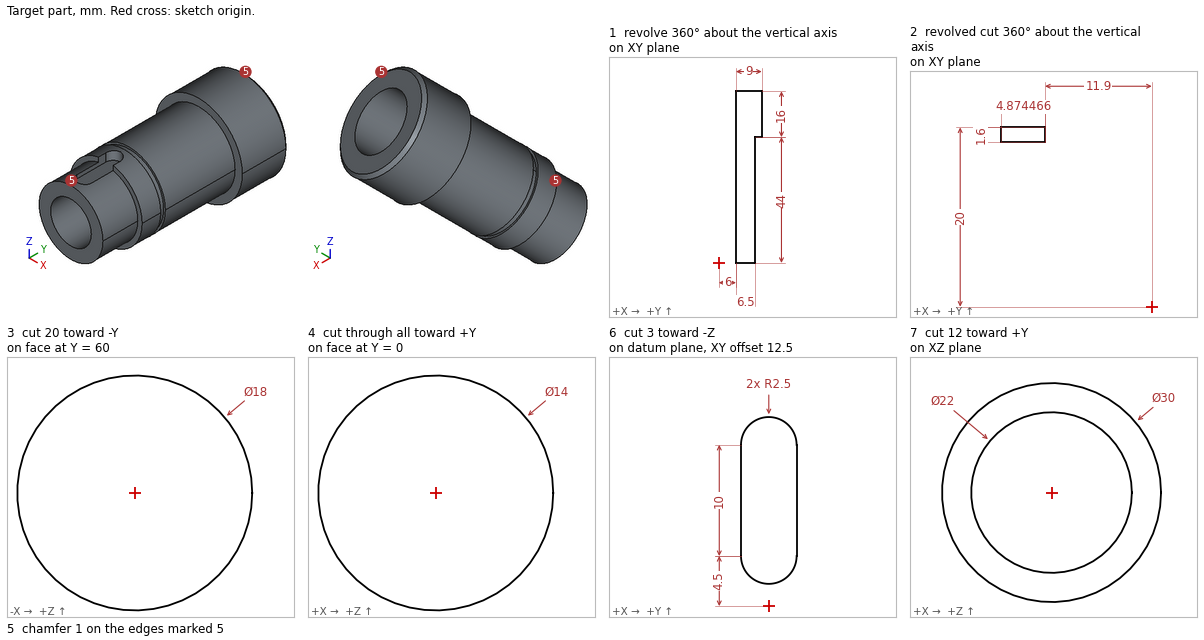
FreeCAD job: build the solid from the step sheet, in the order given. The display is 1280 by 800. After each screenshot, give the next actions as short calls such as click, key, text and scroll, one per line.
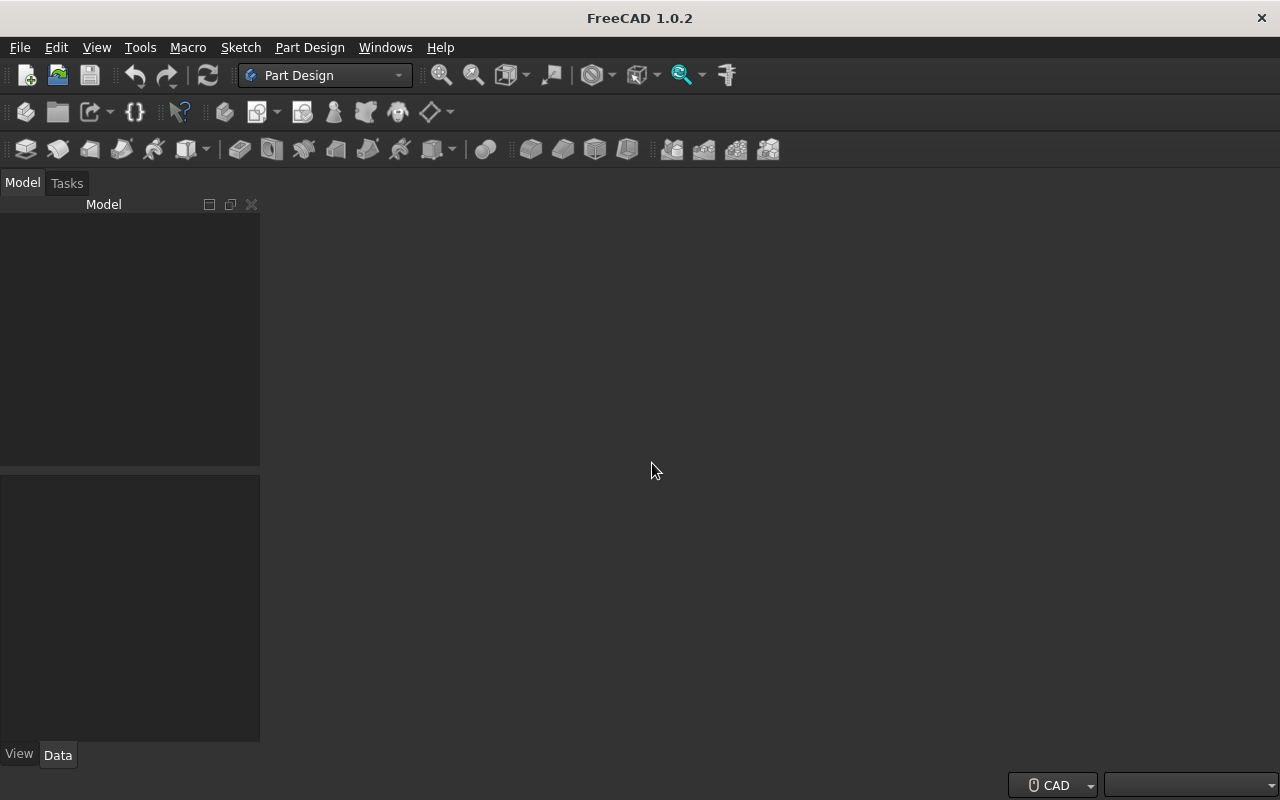
click(26, 76)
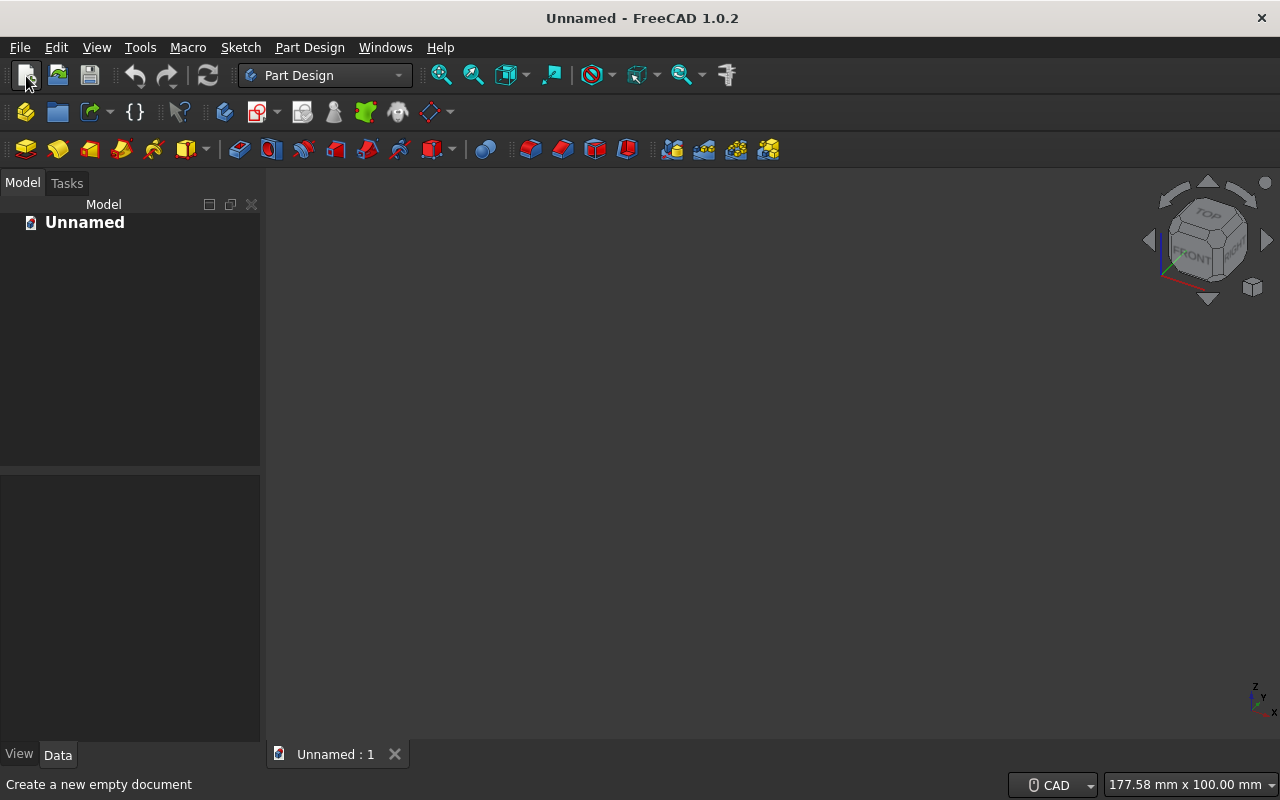
click(258, 112)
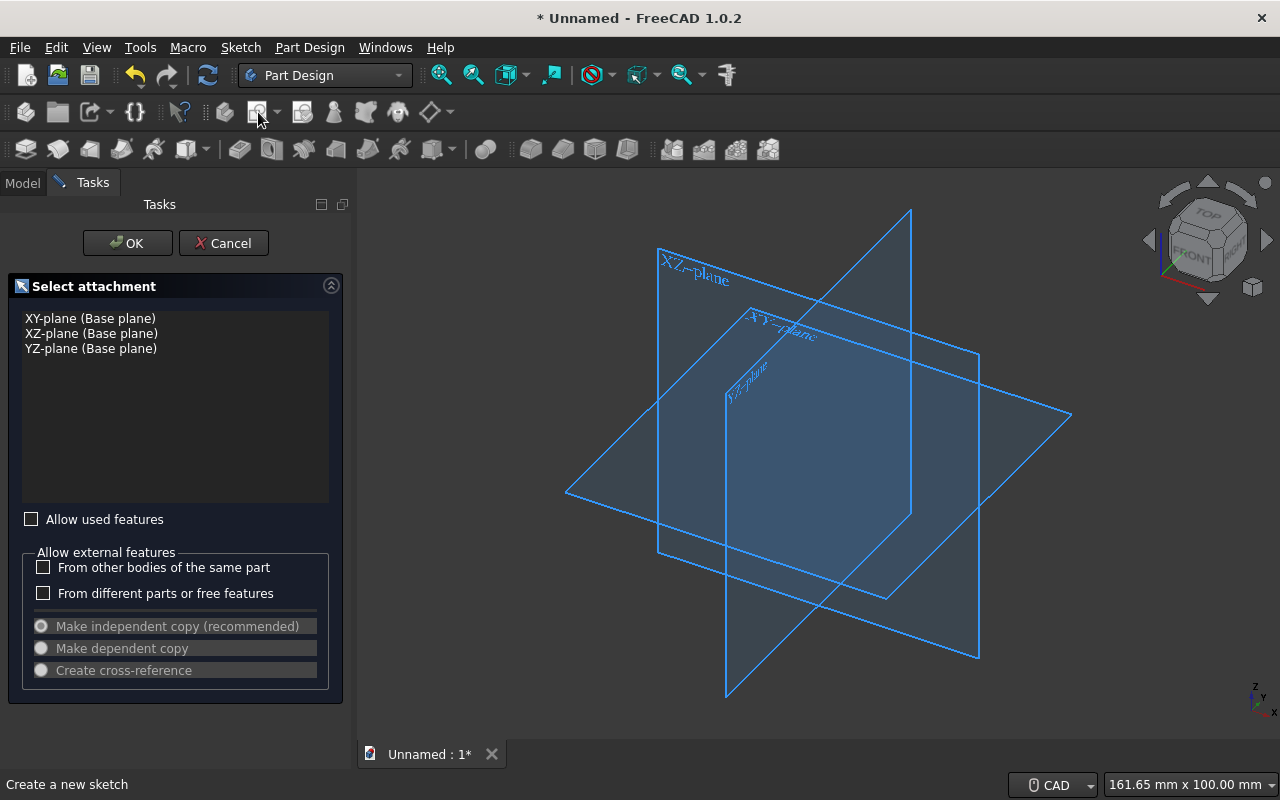
click(82, 318)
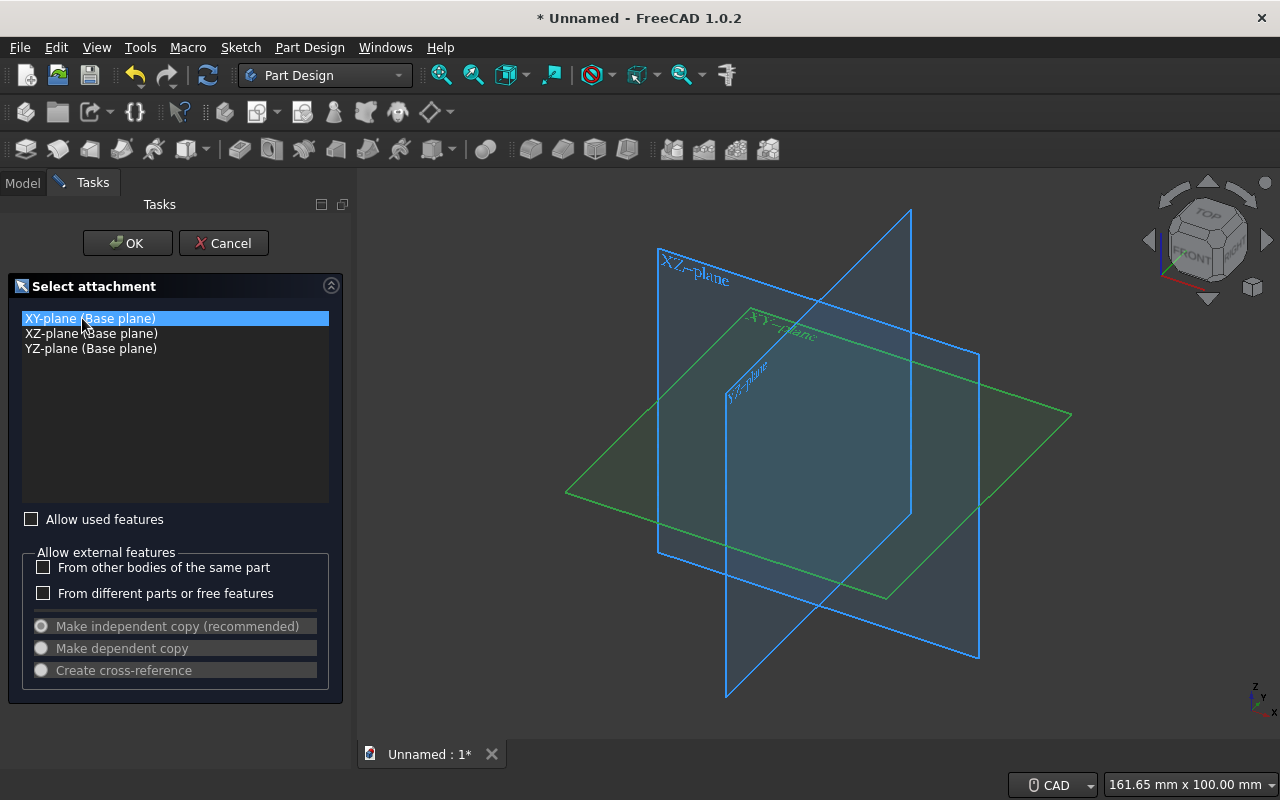
click(128, 243)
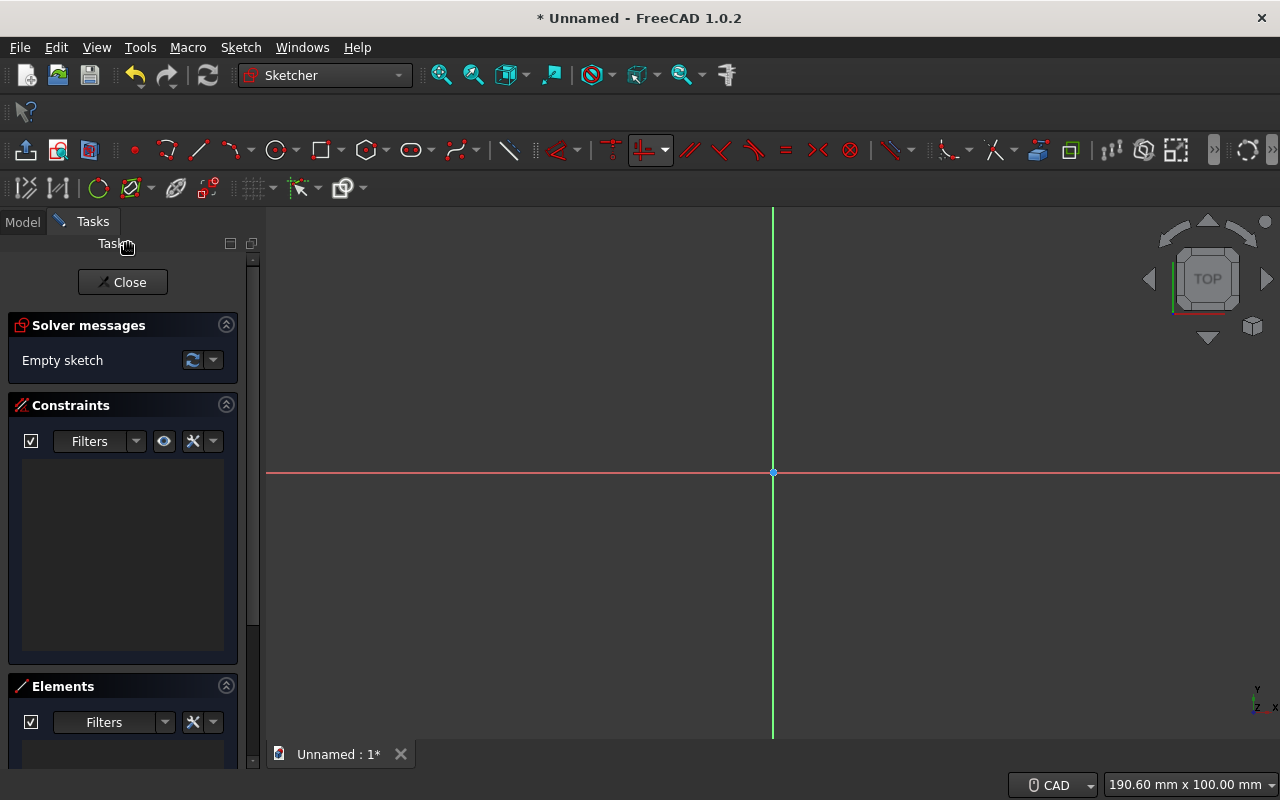
scroll(484, 711, down, 2)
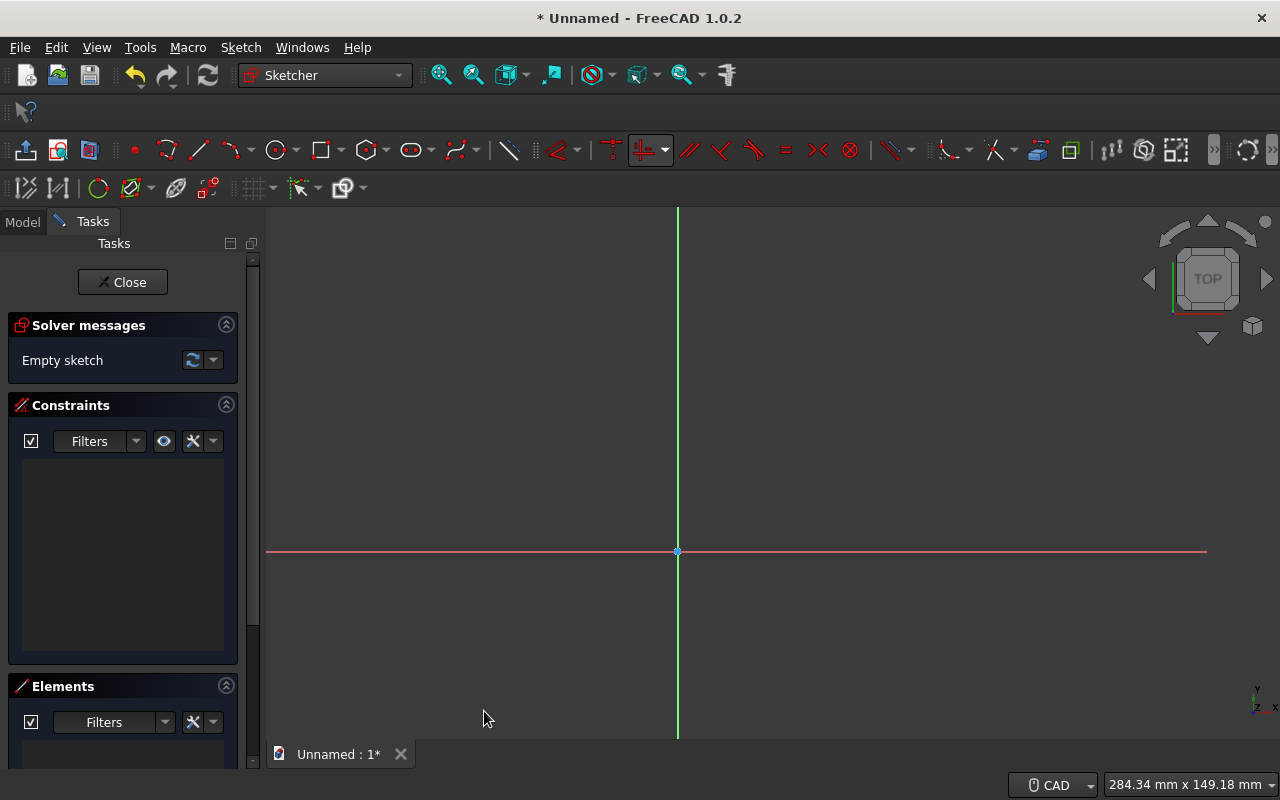
scroll(705, 387, up, 2)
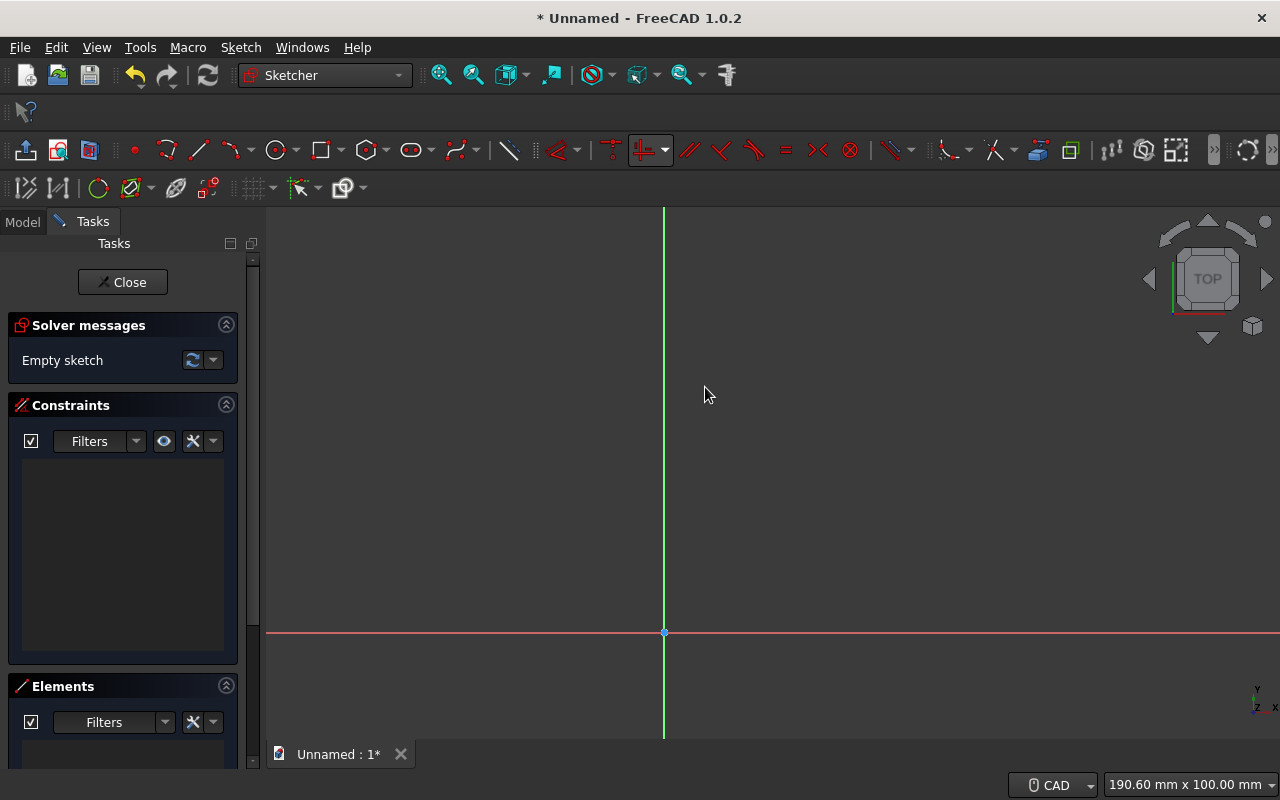
click(168, 150)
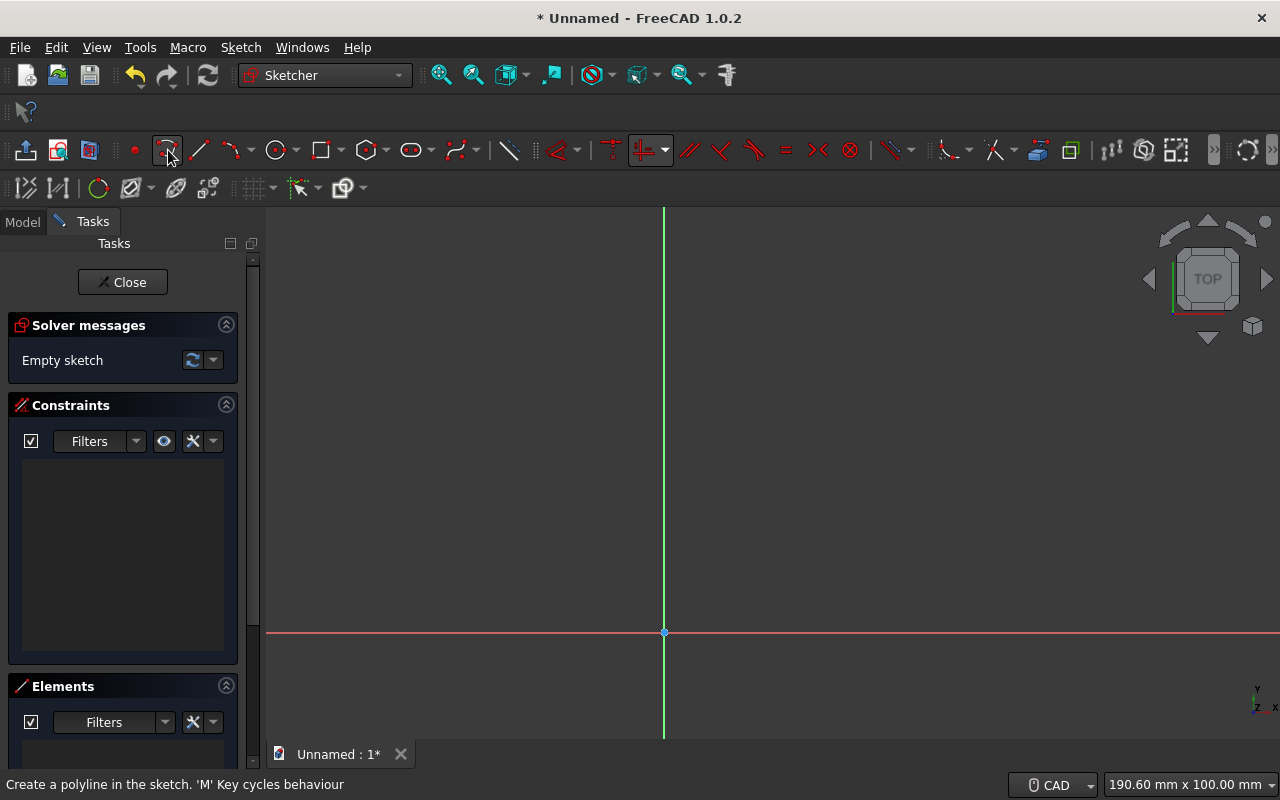
click(696, 633)
click(731, 624)
click(731, 399)
click(744, 399)
click(744, 313)
click(696, 313)
click(696, 633)
key(Escape)
key(Escape)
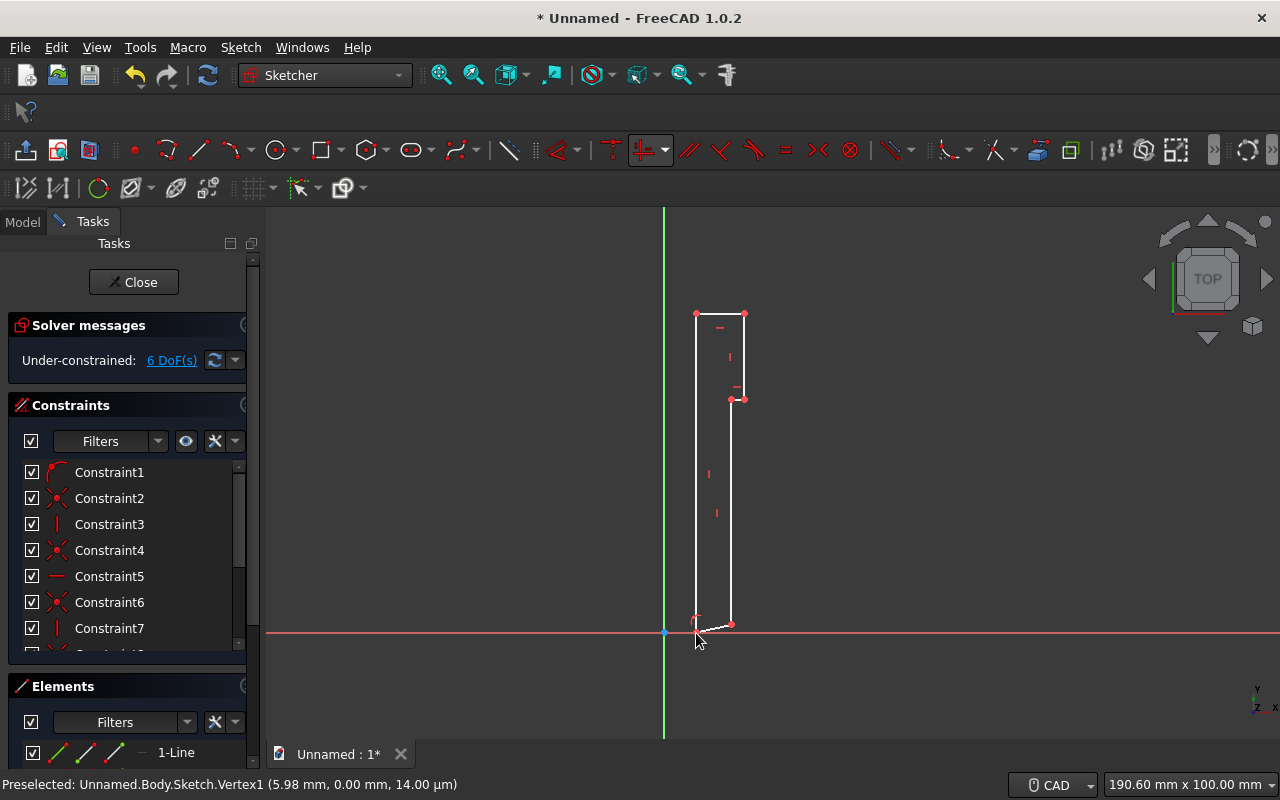
scroll(707, 630, up, 2)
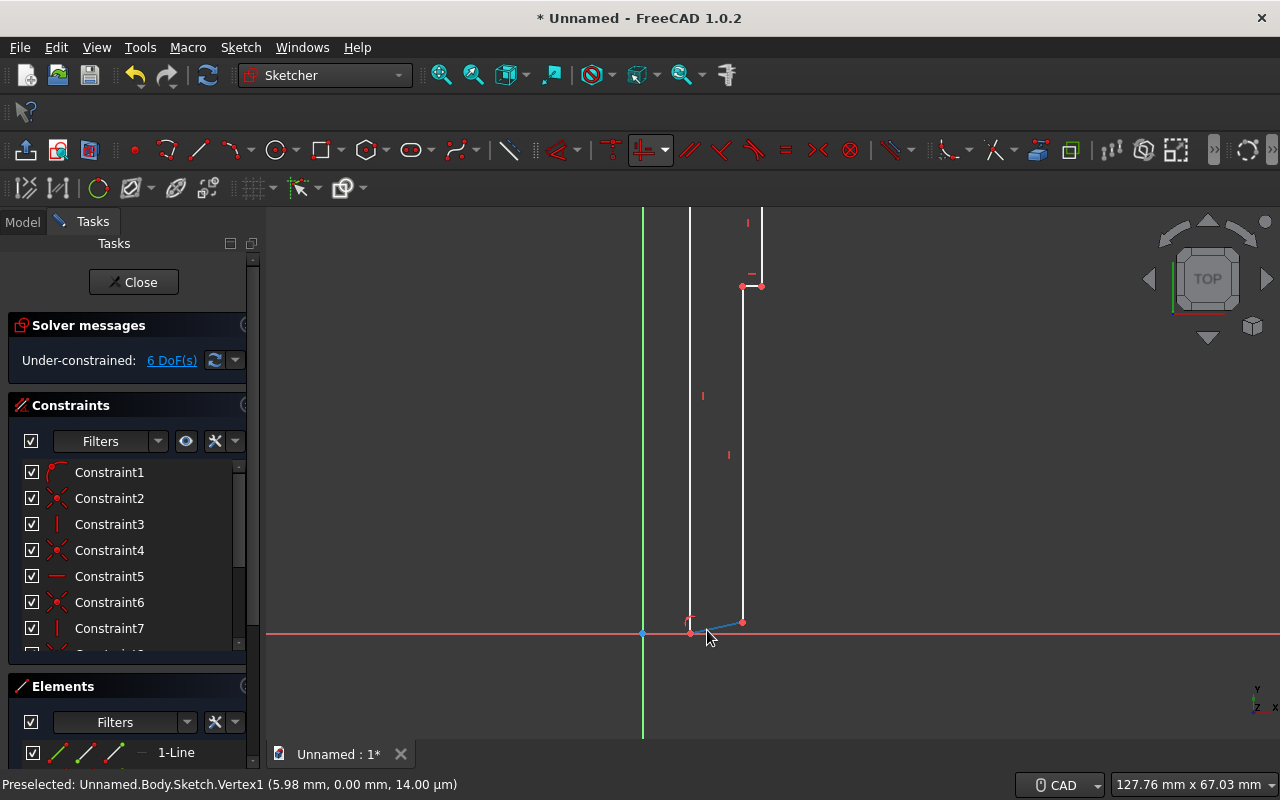
click(706, 630)